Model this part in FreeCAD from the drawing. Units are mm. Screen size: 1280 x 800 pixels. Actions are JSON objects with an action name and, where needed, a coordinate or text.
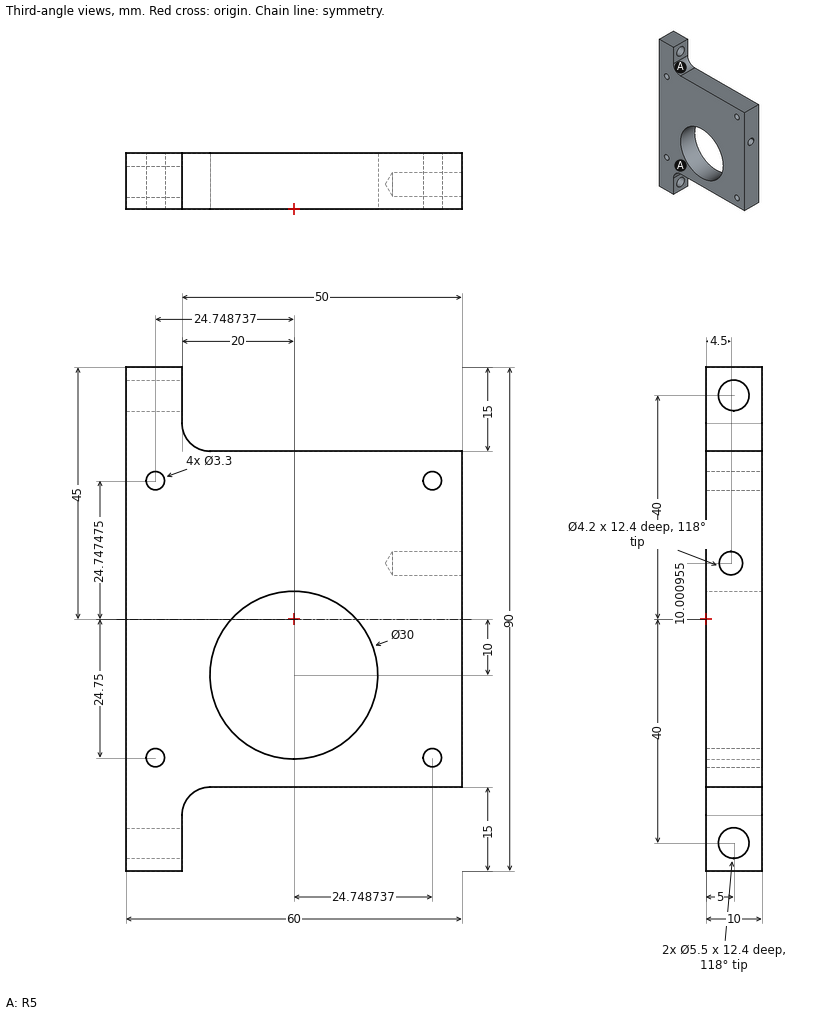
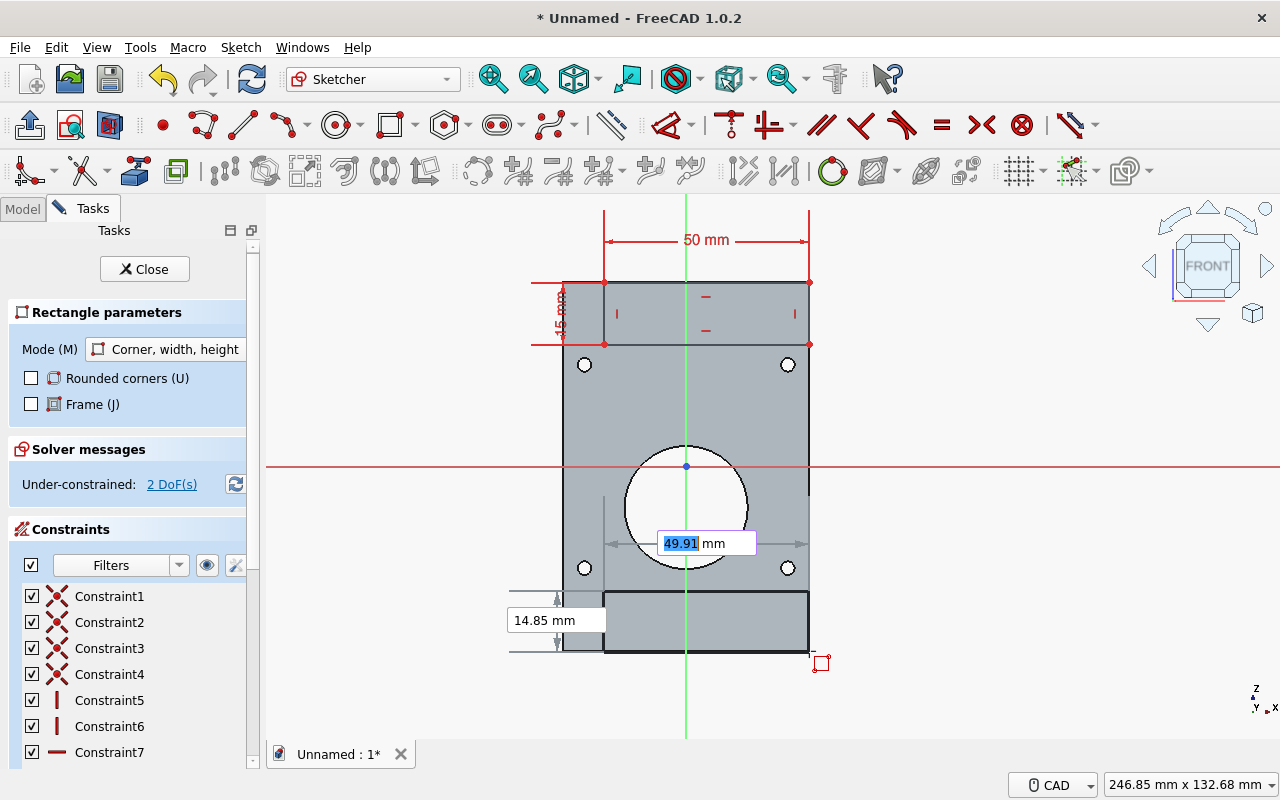
{"action": "type", "text": "50"}
{"action": "key", "text": "Tab"}
{"action": "type", "text": "15"}
{"action": "key", "text": "Return"}
{"action": "key", "text": "Escape"}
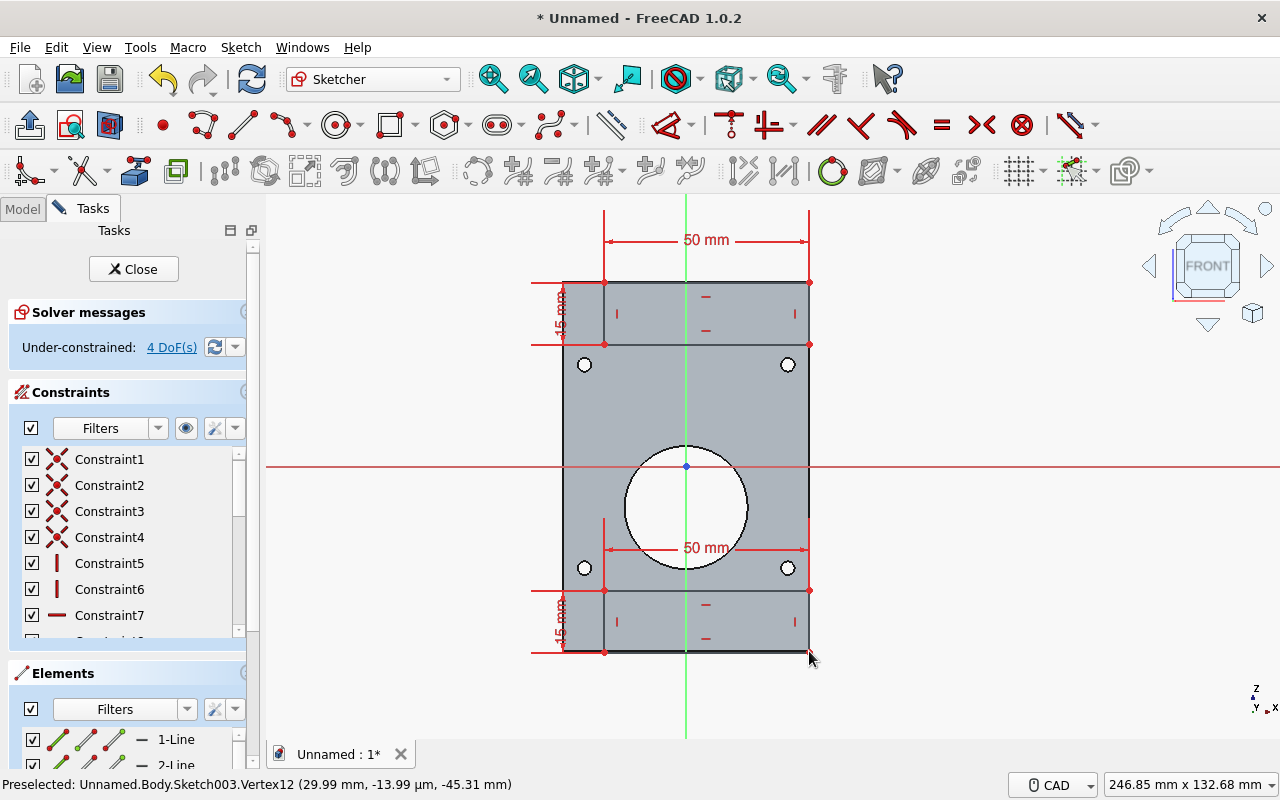
{"action": "left_click", "coordinate": [604, 345]}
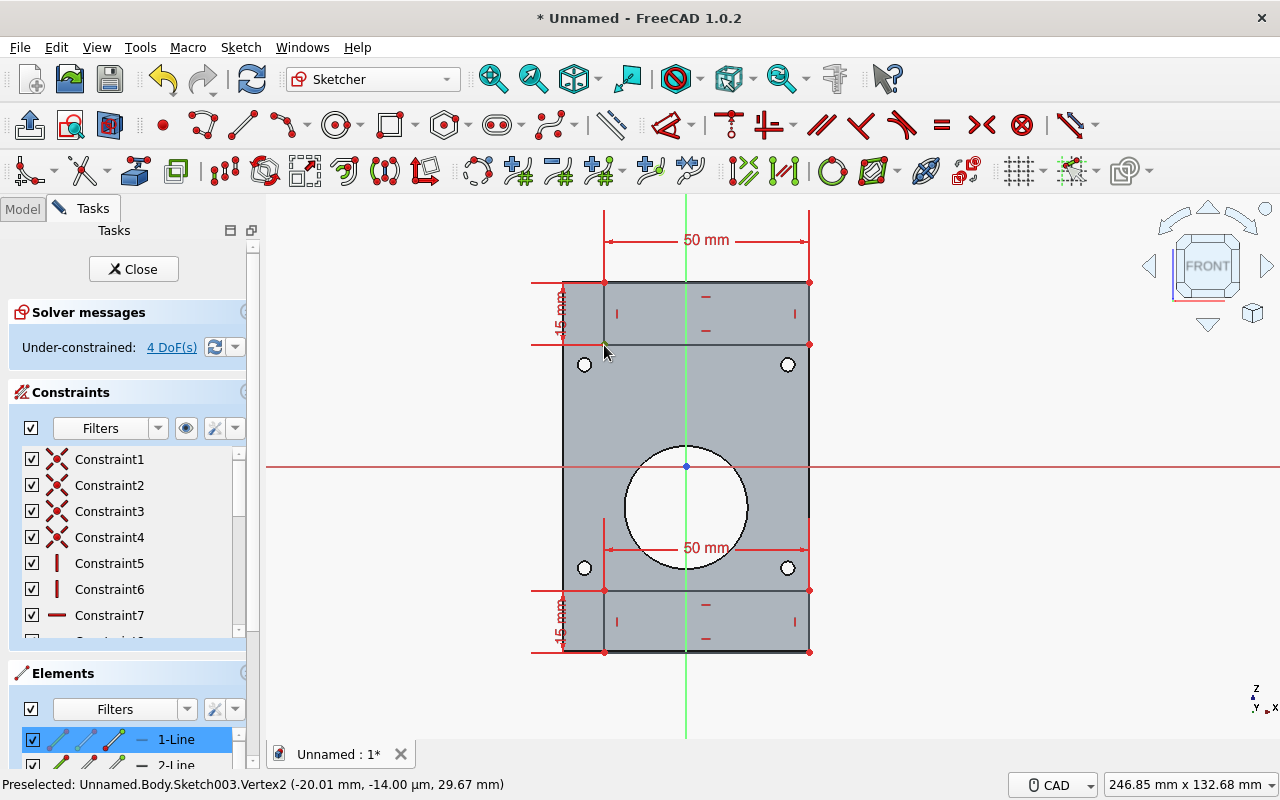
{"action": "left_click", "coordinate": [604, 591]}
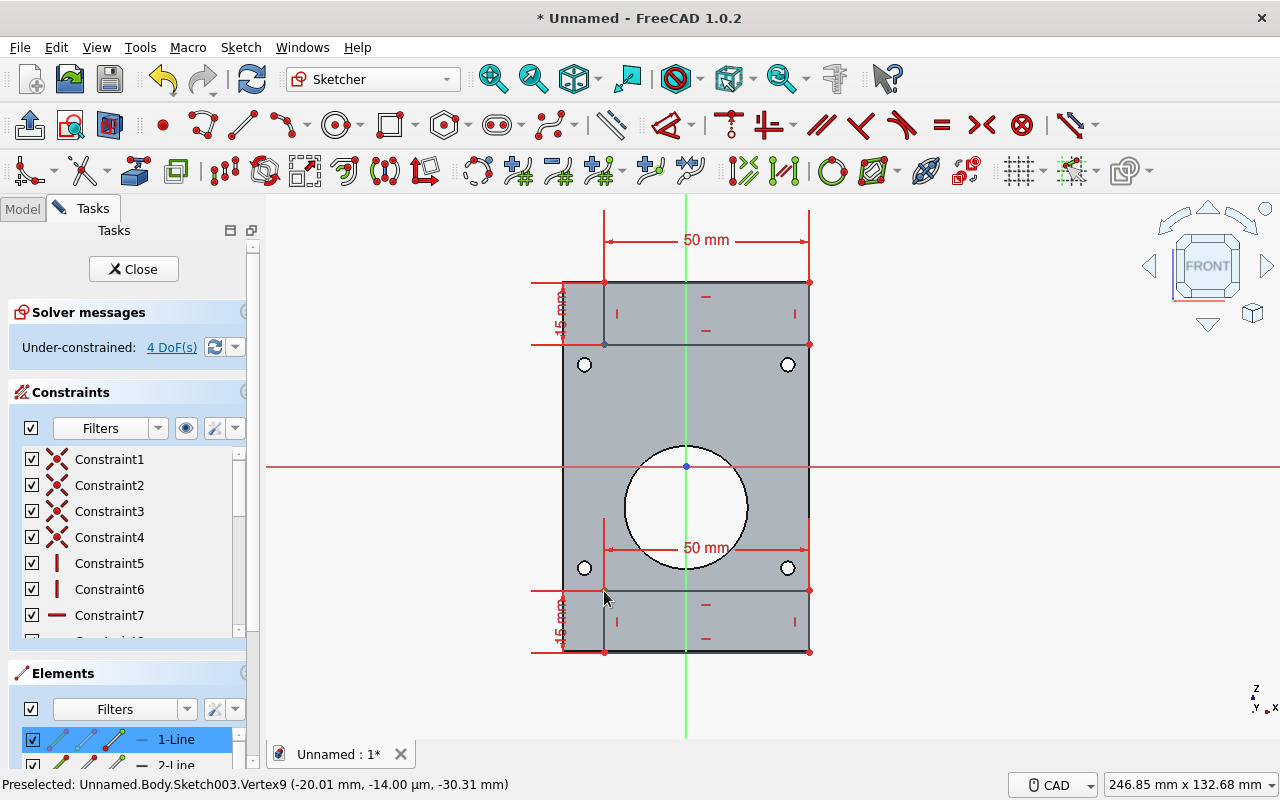
{"action": "left_click", "coordinate": [353, 467]}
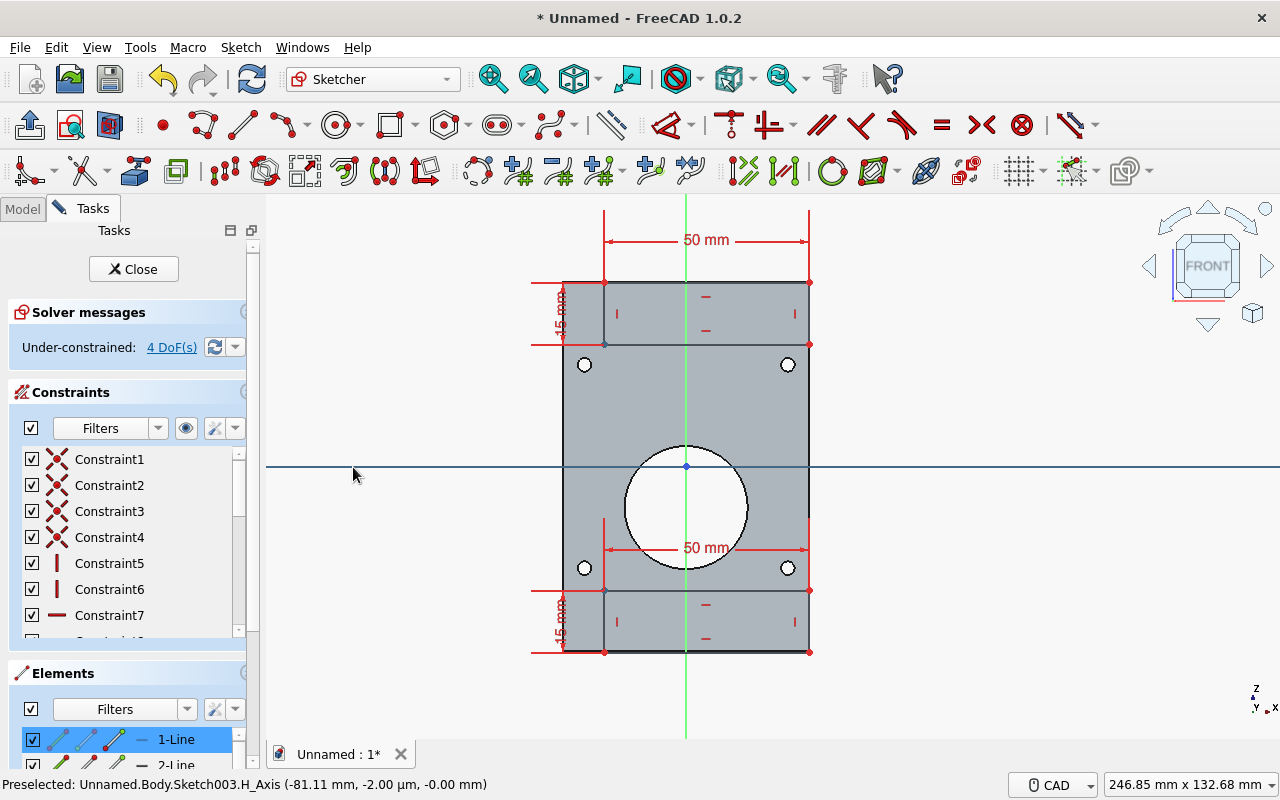
{"action": "key", "text": "s"}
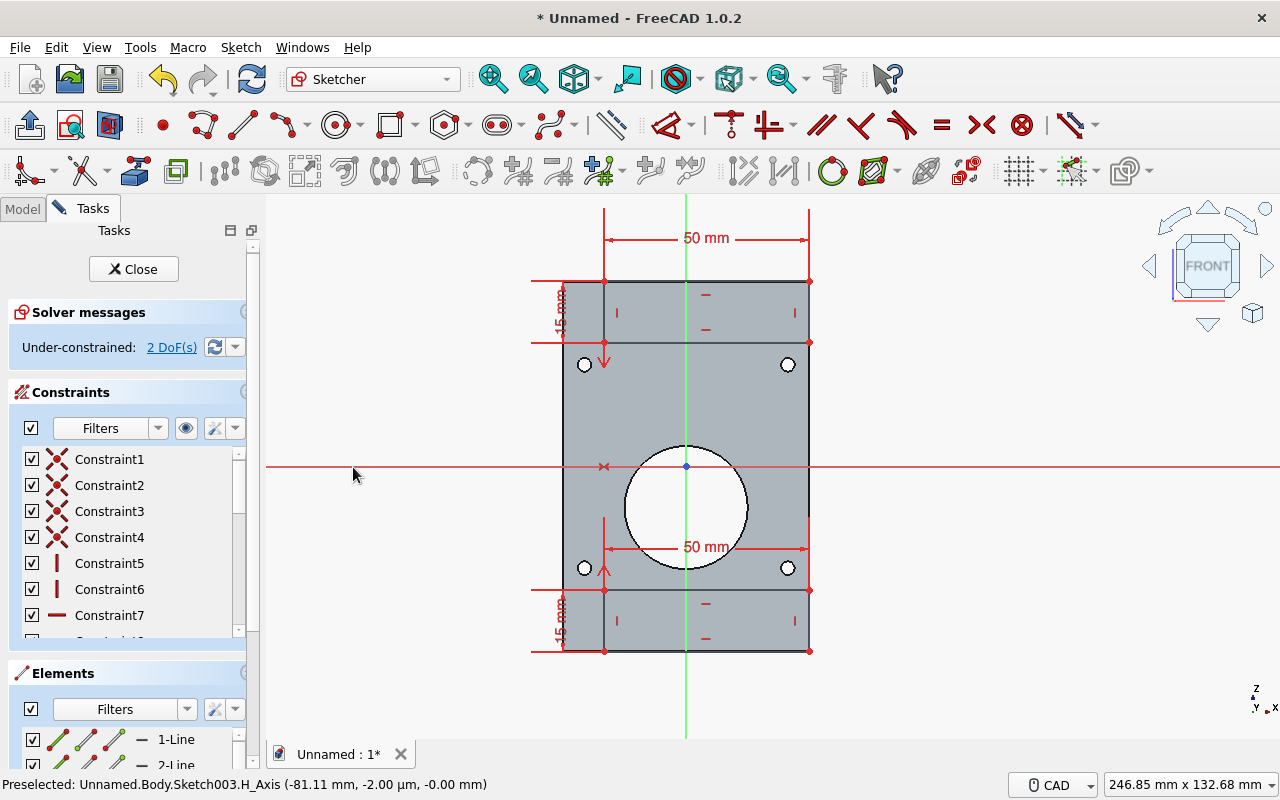
{"action": "key", "text": "d"}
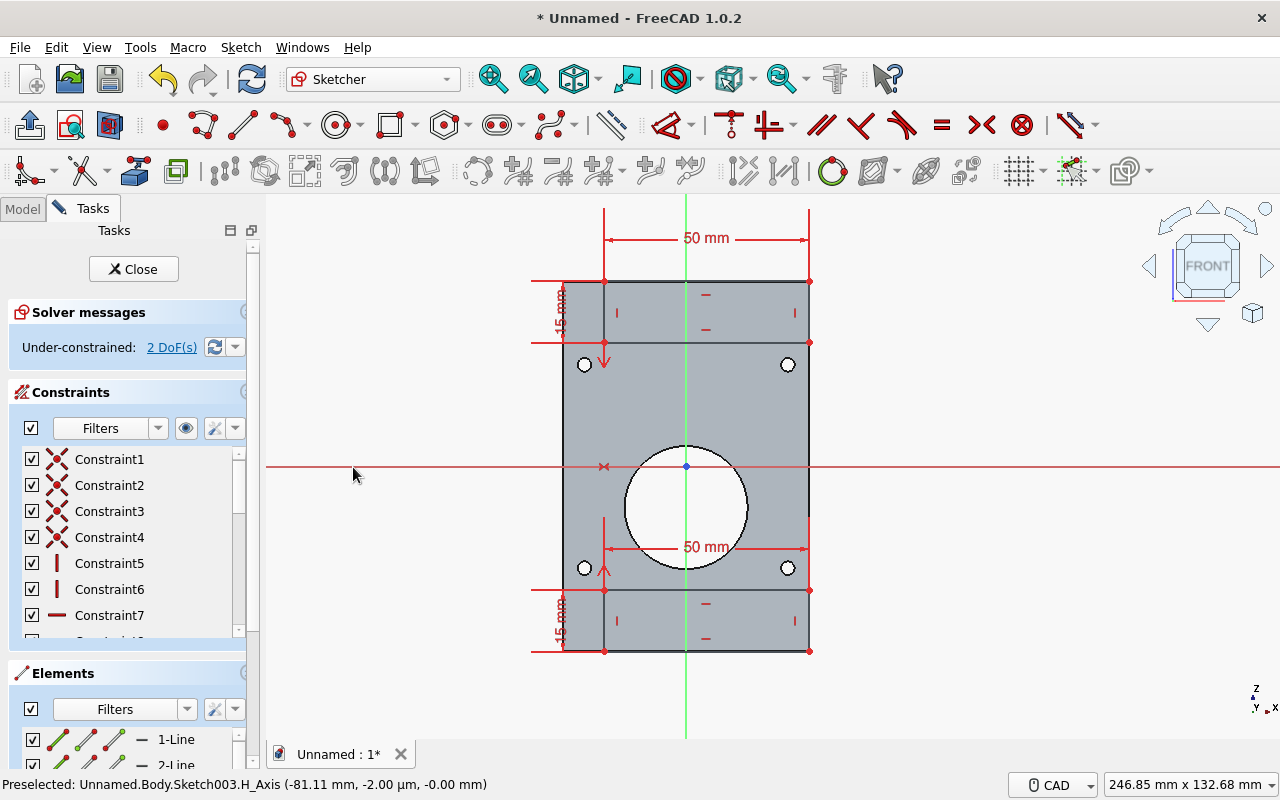
{"action": "left_click", "coordinate": [604, 281]}
{"action": "left_click", "coordinate": [645, 247]}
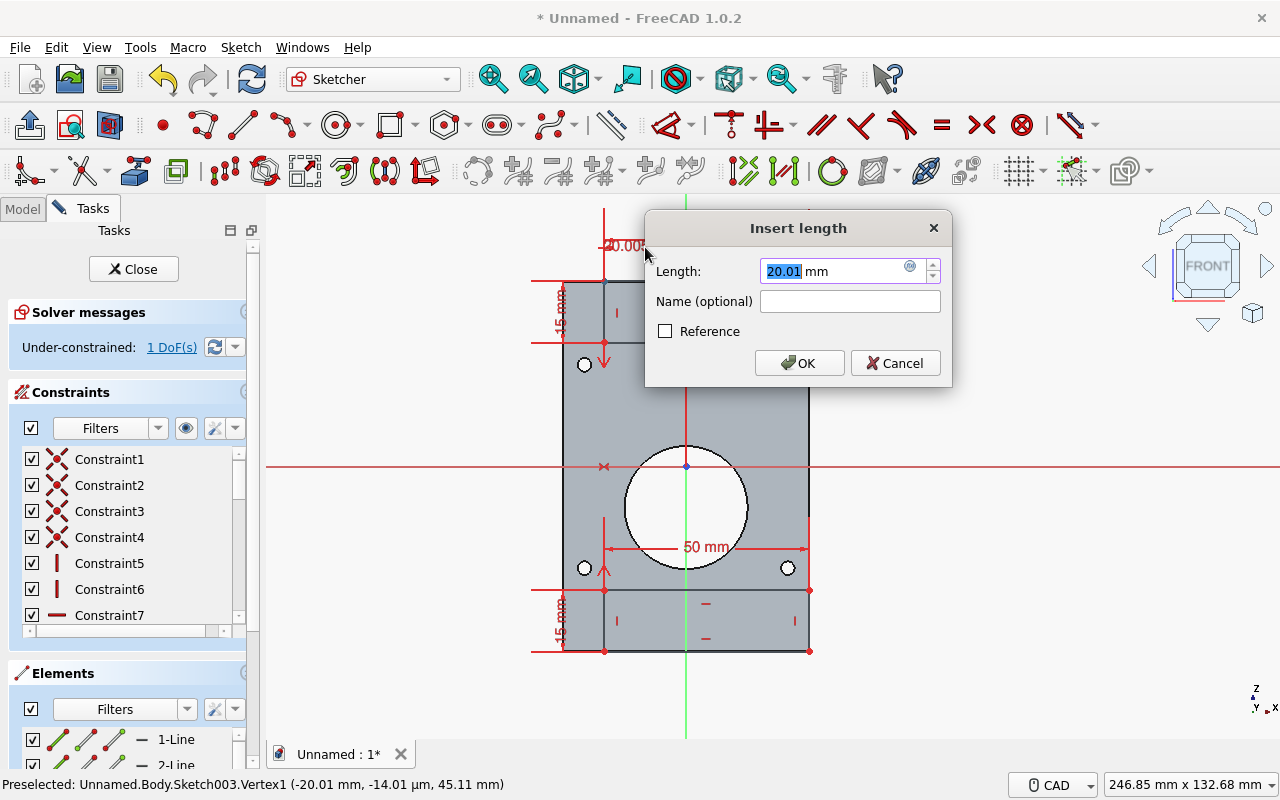
{"action": "type", "text": "20"}
{"action": "key", "text": "Return"}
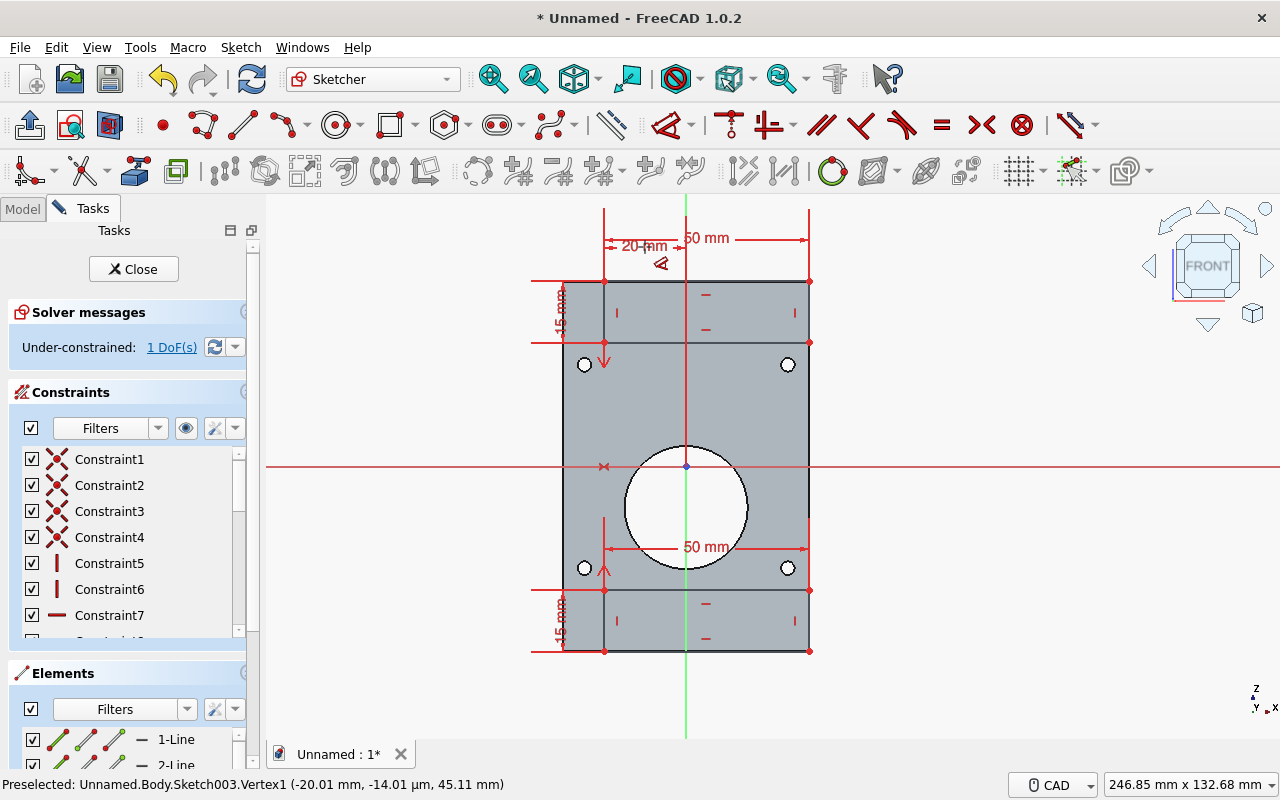
{"action": "left_click", "coordinate": [604, 281]}
{"action": "left_click", "coordinate": [570, 374]}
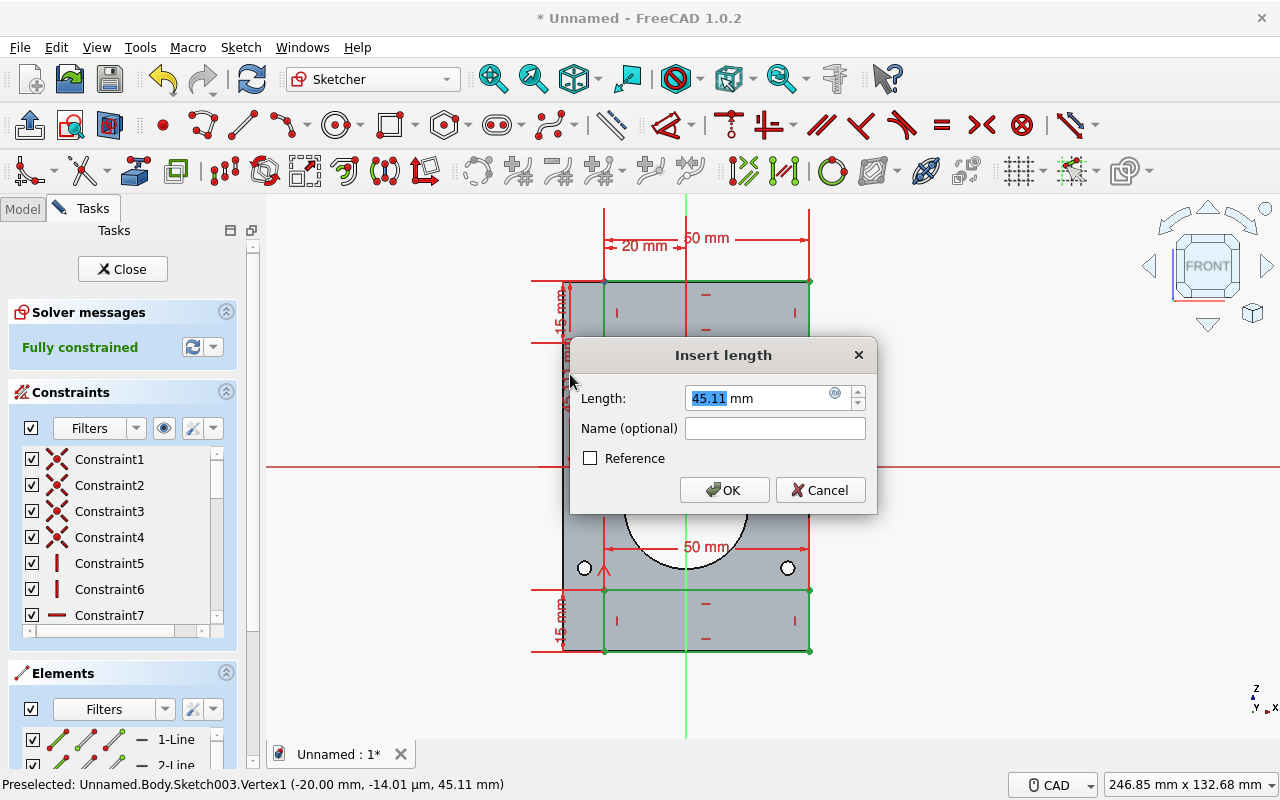
{"action": "type", "text": "45"}
{"action": "key", "text": "Return"}
{"action": "key", "text": "Escape"}